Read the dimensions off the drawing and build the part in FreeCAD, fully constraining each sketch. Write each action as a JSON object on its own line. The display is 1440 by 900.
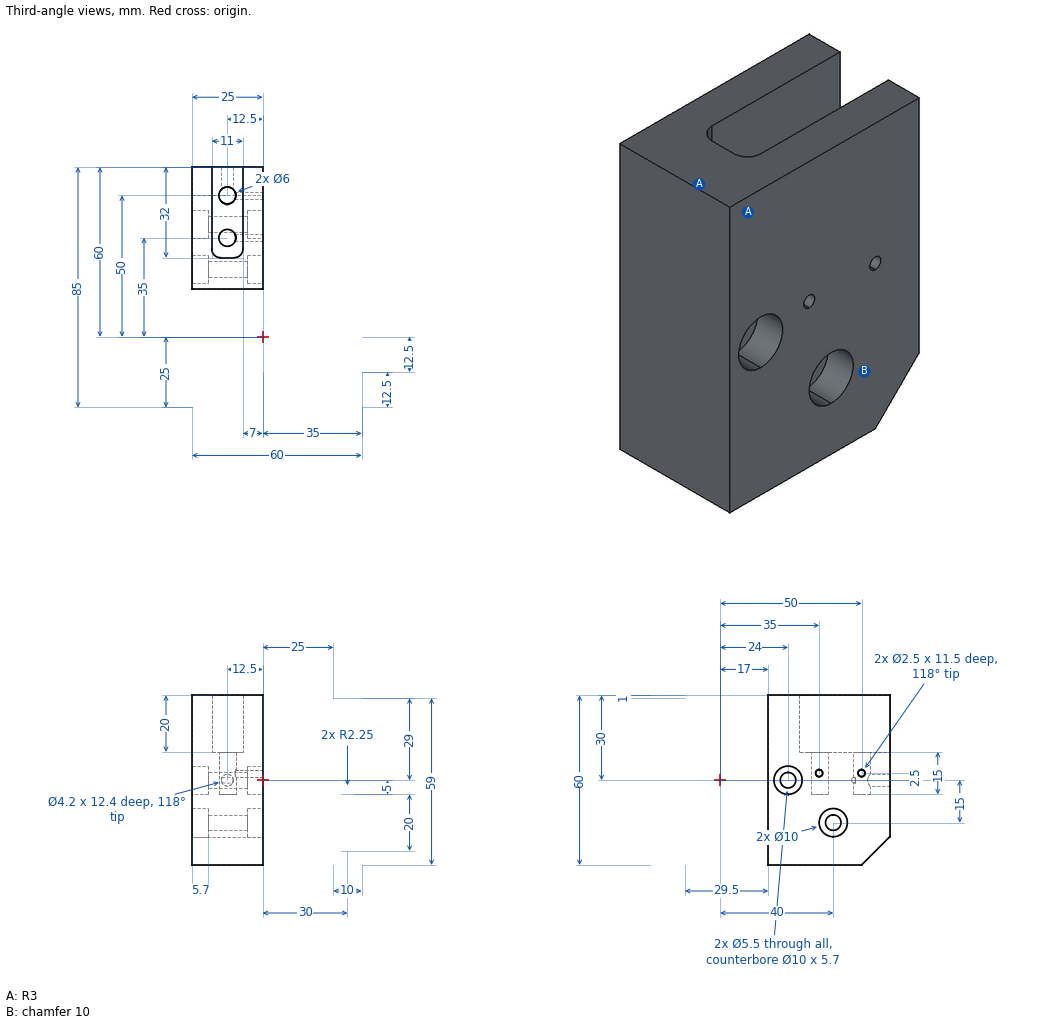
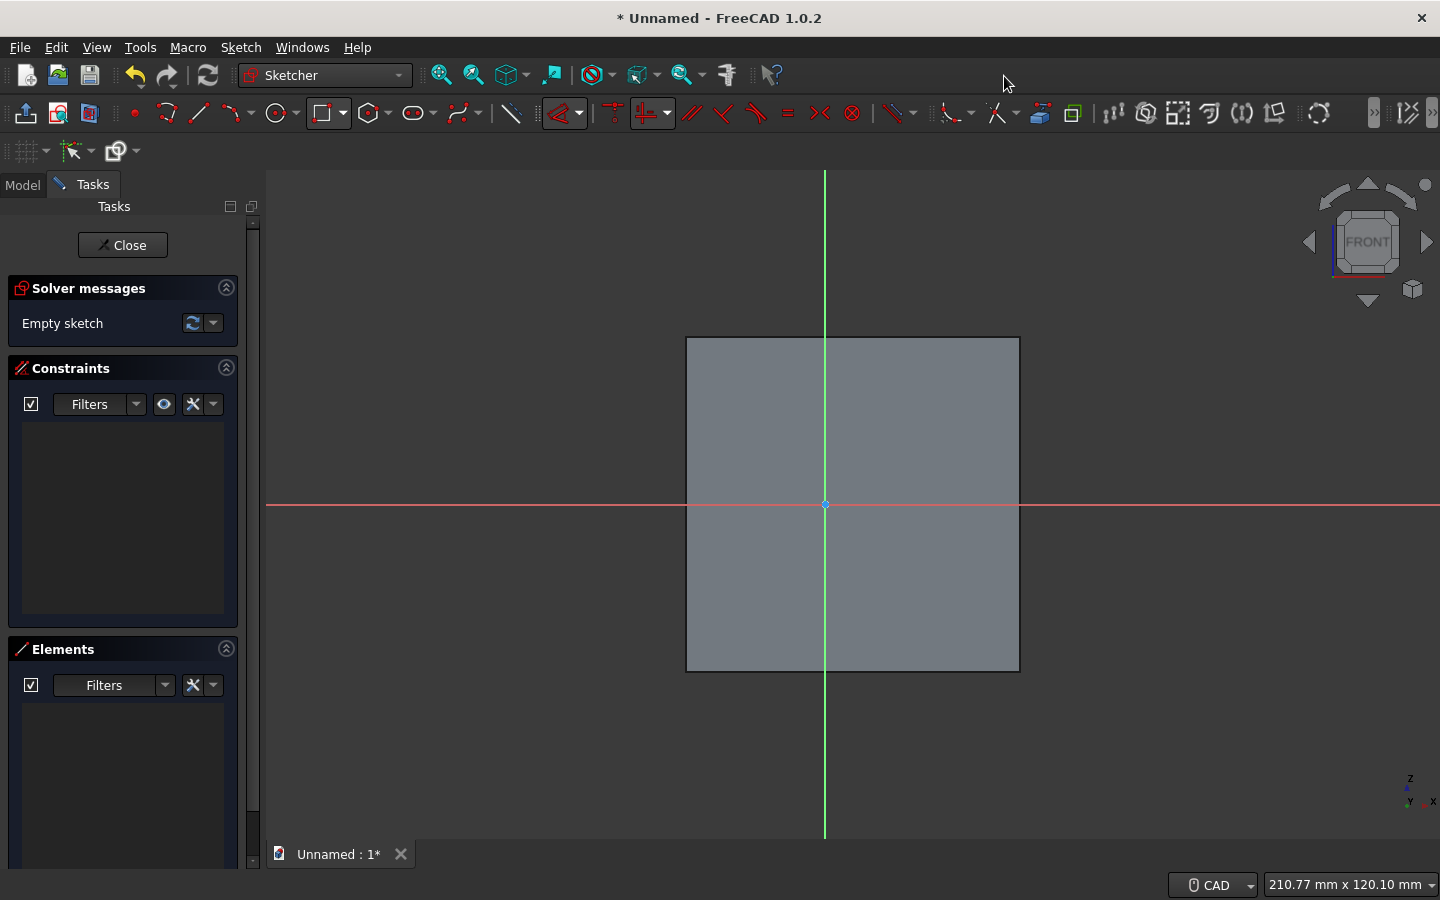
{"action": "scroll", "coordinate": [991, 625], "scroll_direction": "up", "scroll_amount": 5}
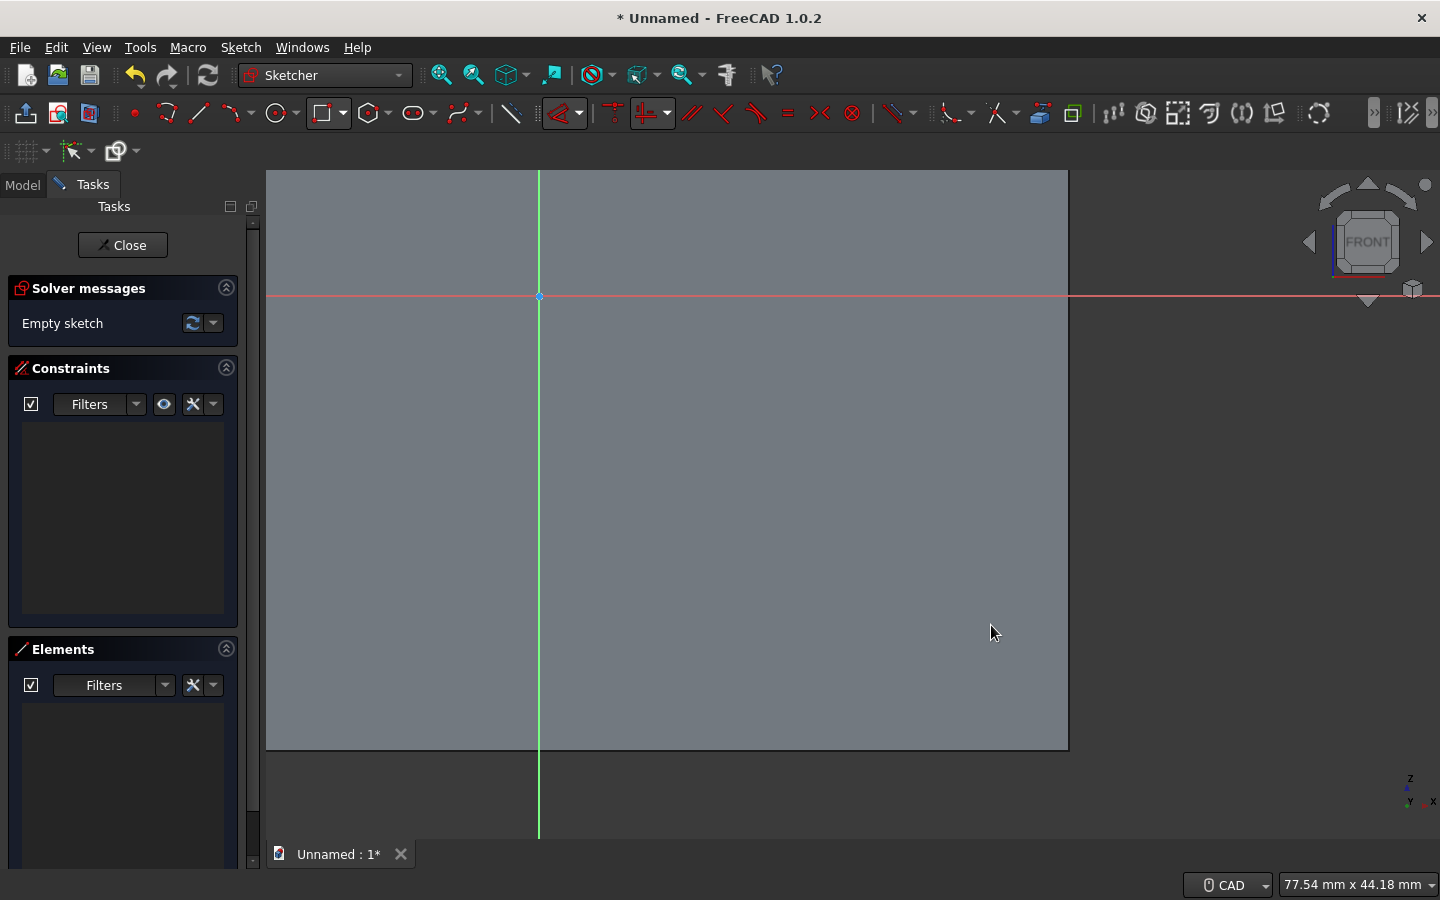
{"action": "left_click", "coordinate": [414, 114]}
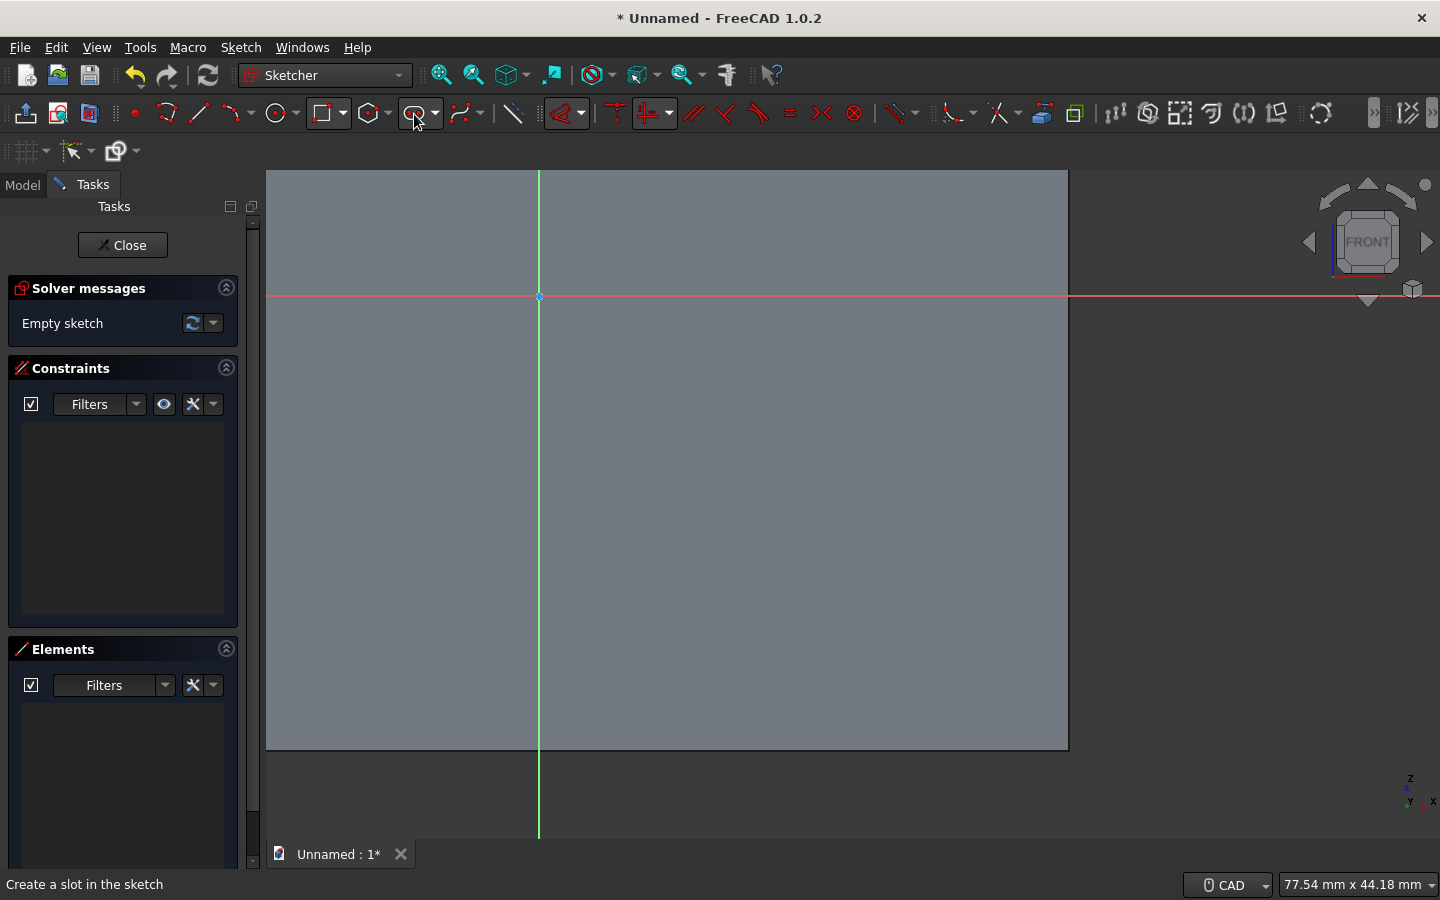
{"action": "left_click", "coordinate": [993, 675]}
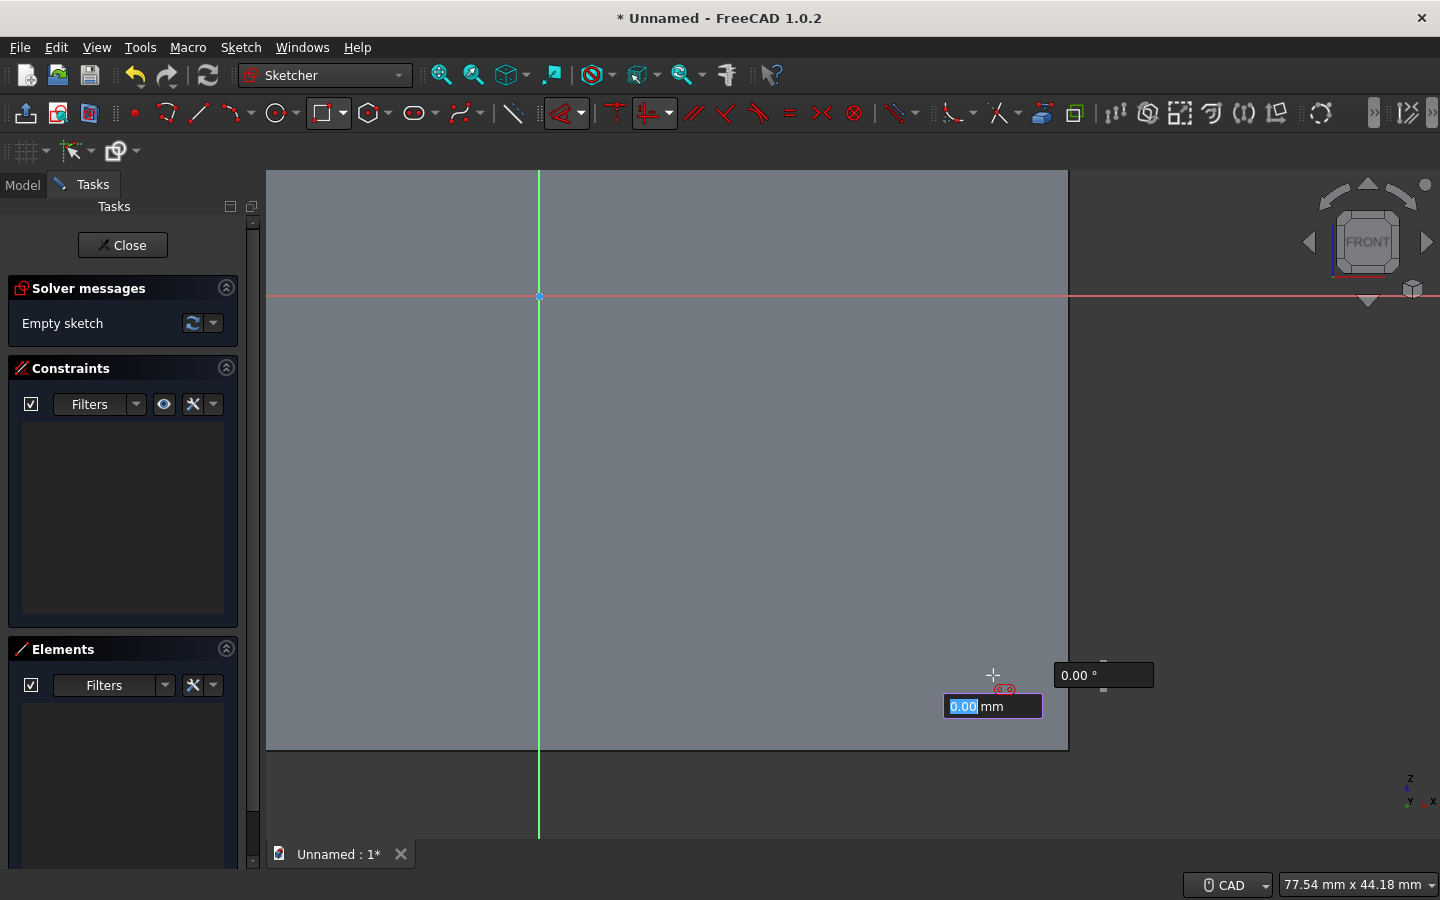
{"action": "left_click", "coordinate": [993, 372]}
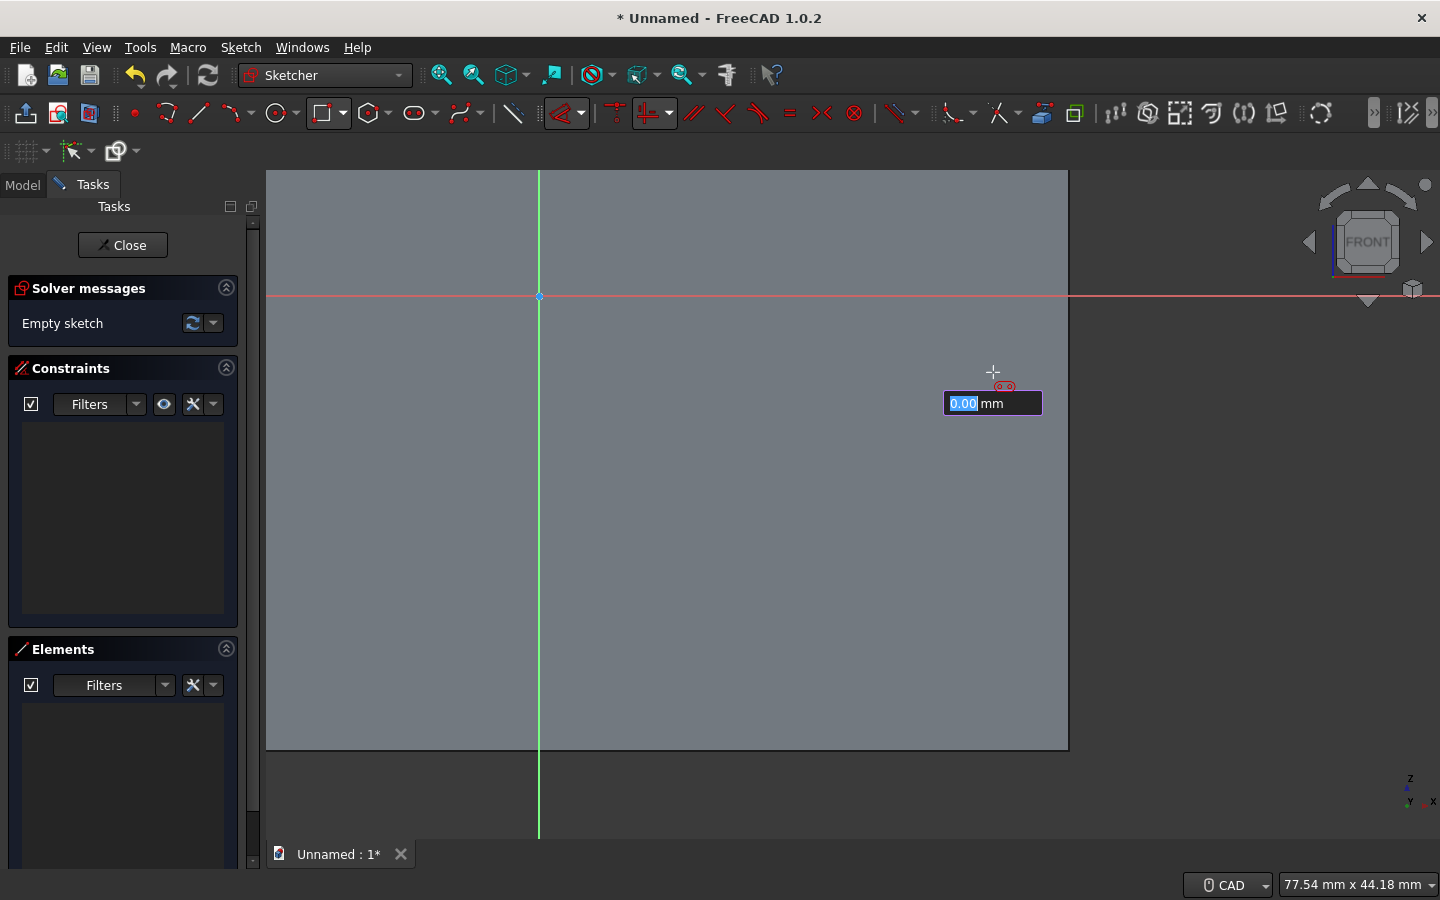
{"action": "left_click", "coordinate": [1027, 523]}
{"action": "key", "text": "Escape"}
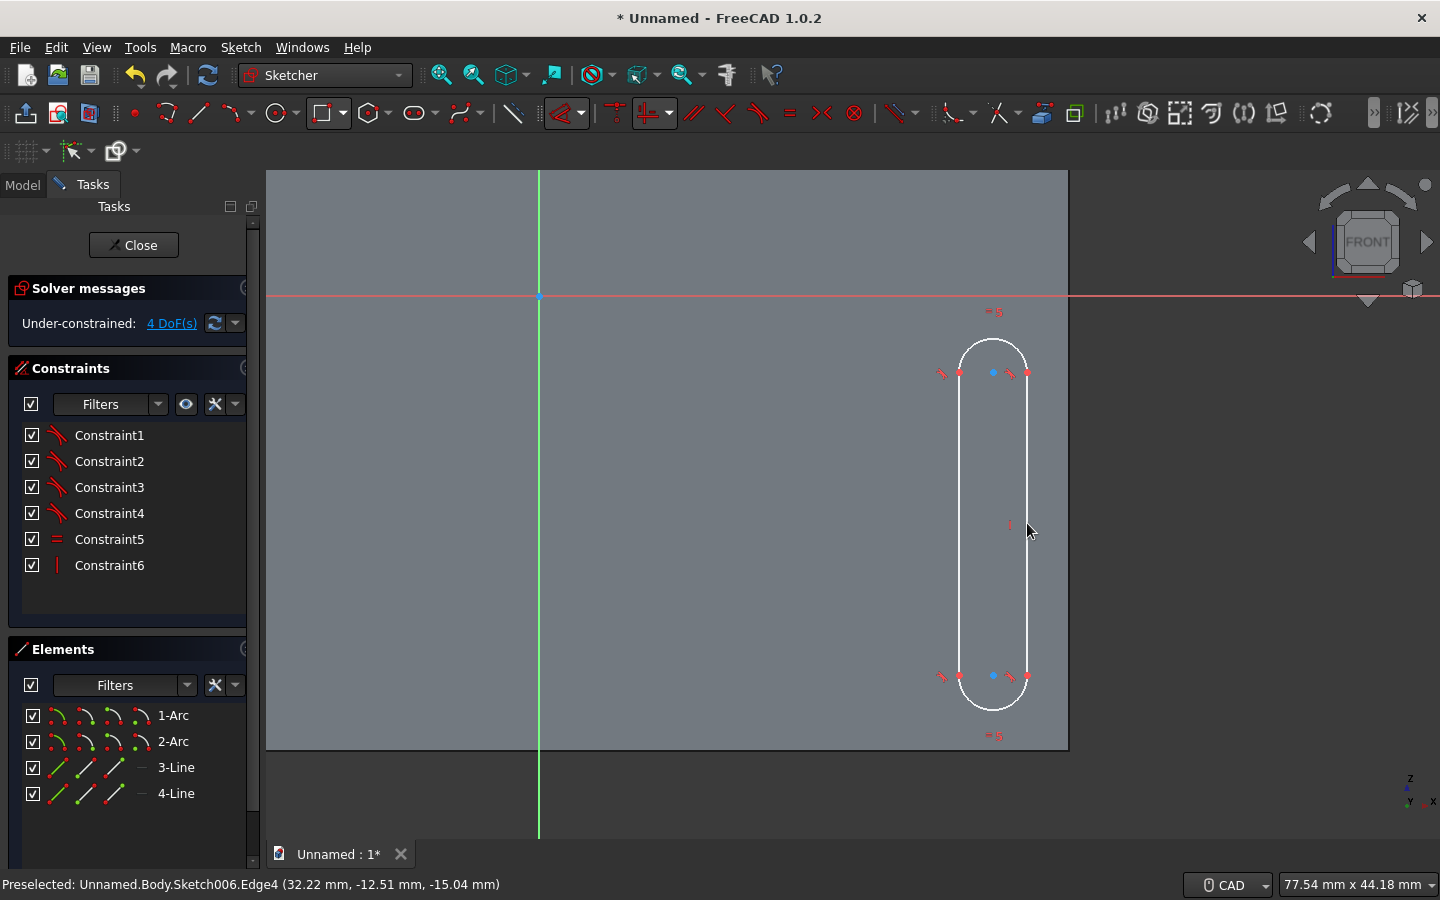
{"action": "left_click", "coordinate": [973, 704]}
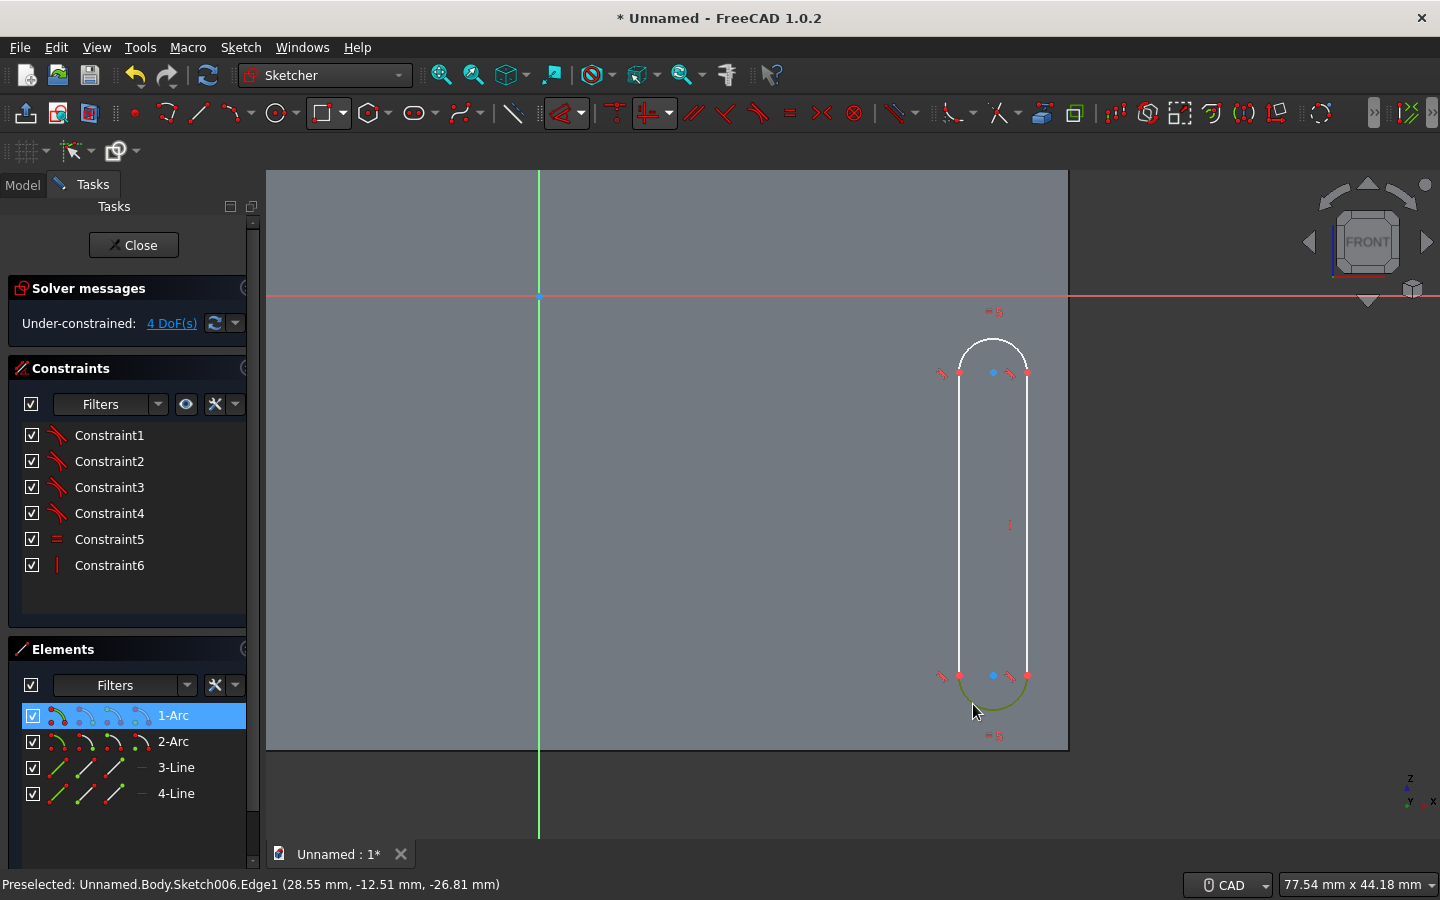
{"action": "key", "text": "k r"}